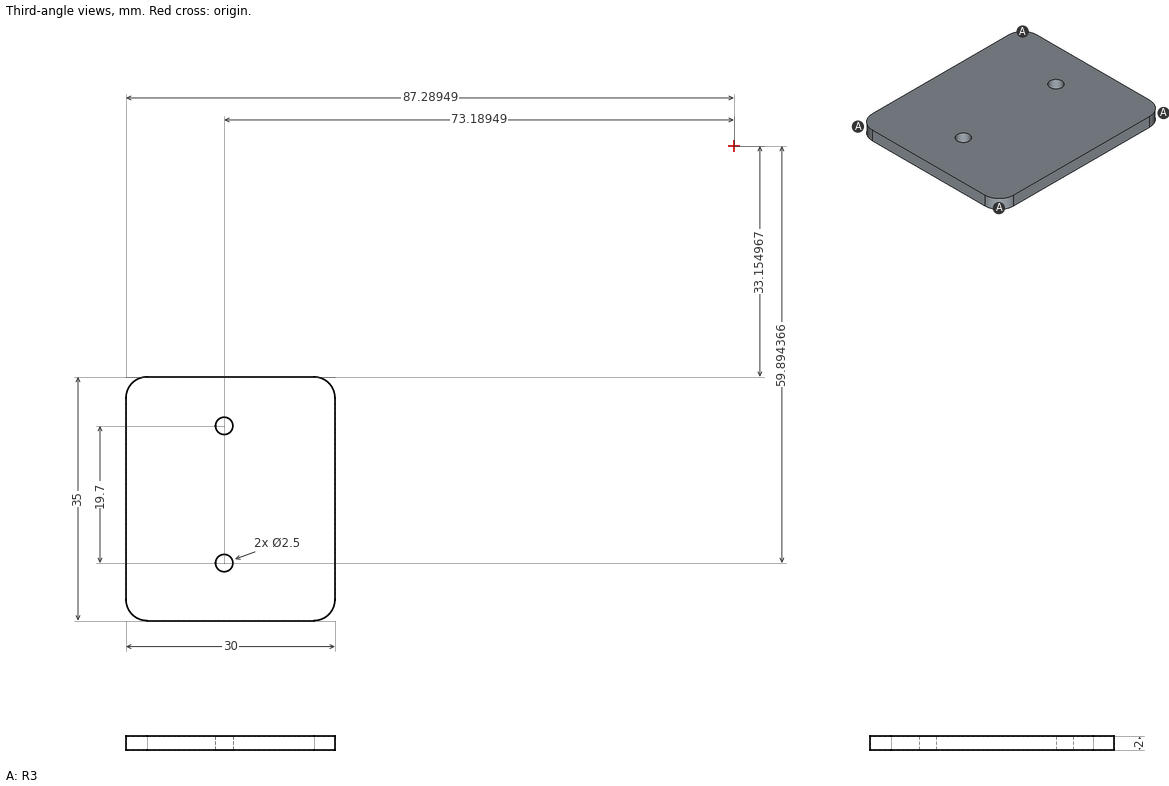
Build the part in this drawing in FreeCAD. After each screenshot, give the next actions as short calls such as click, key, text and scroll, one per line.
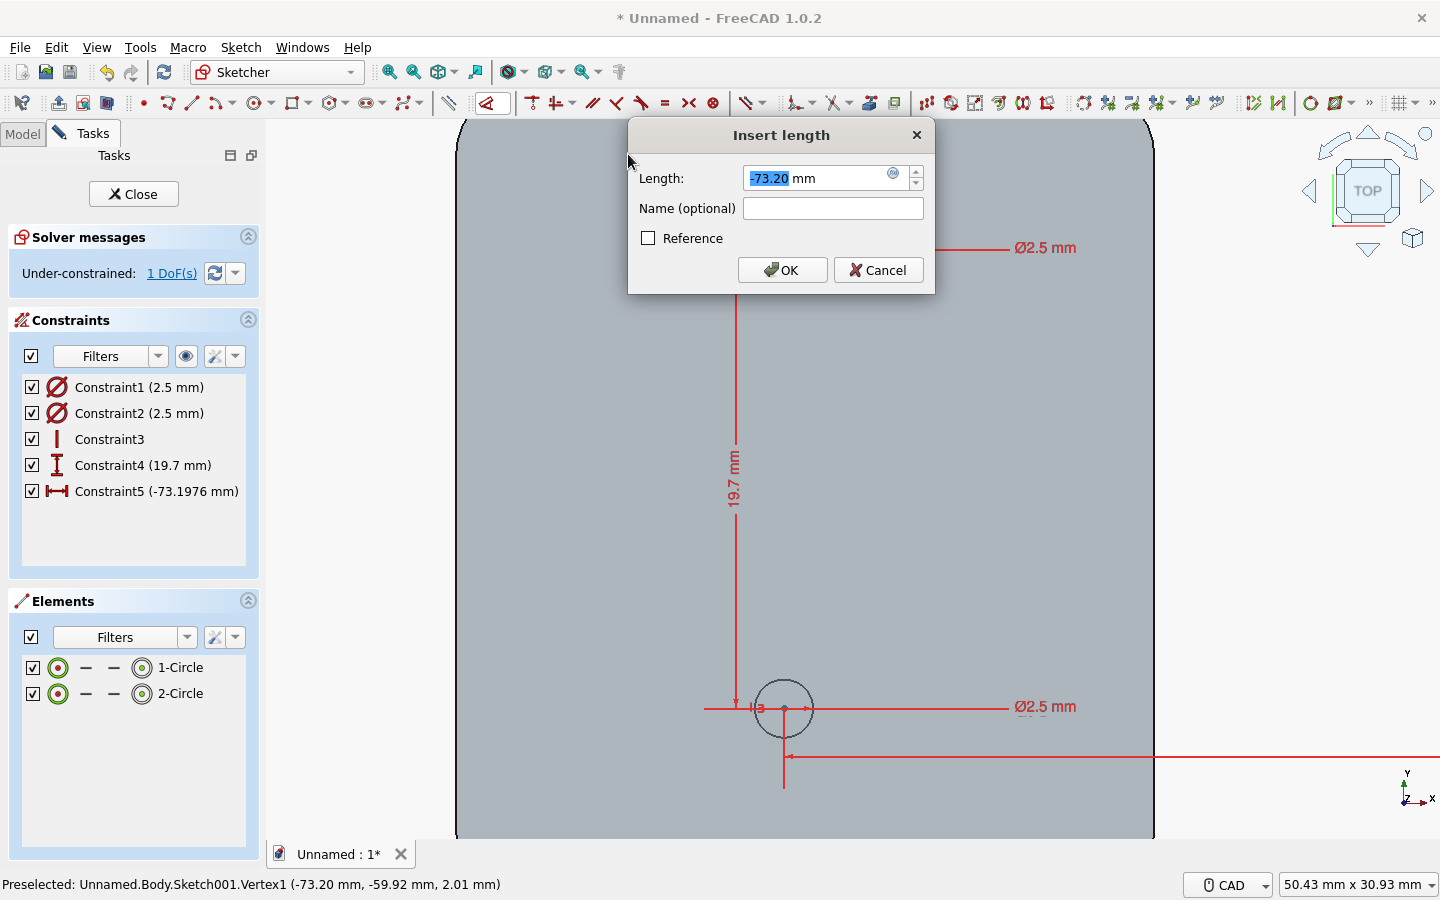
text(-73.18949)
key(Return)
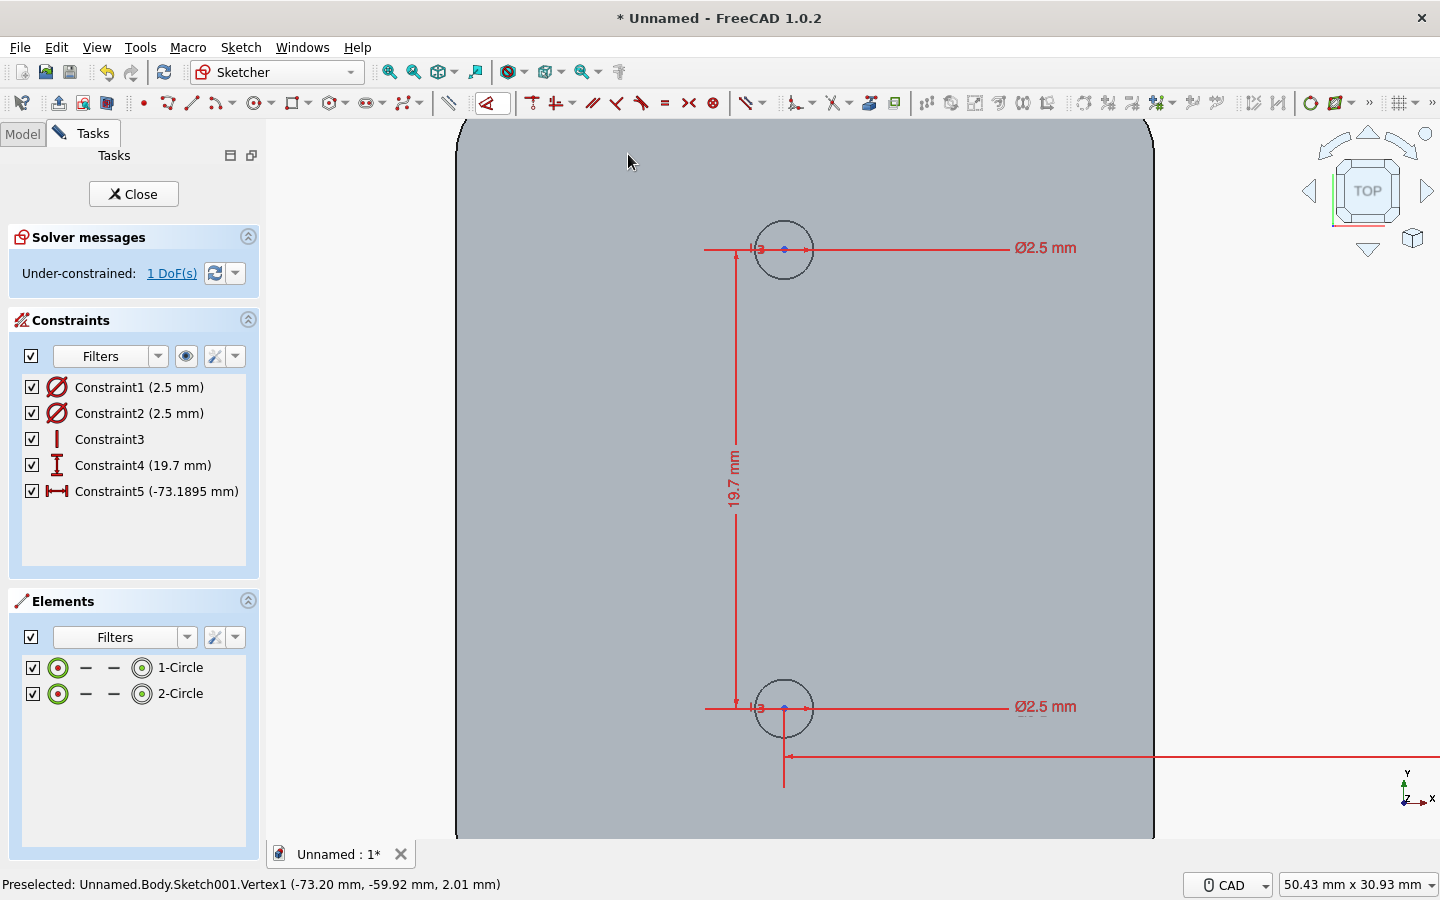
click(784, 709)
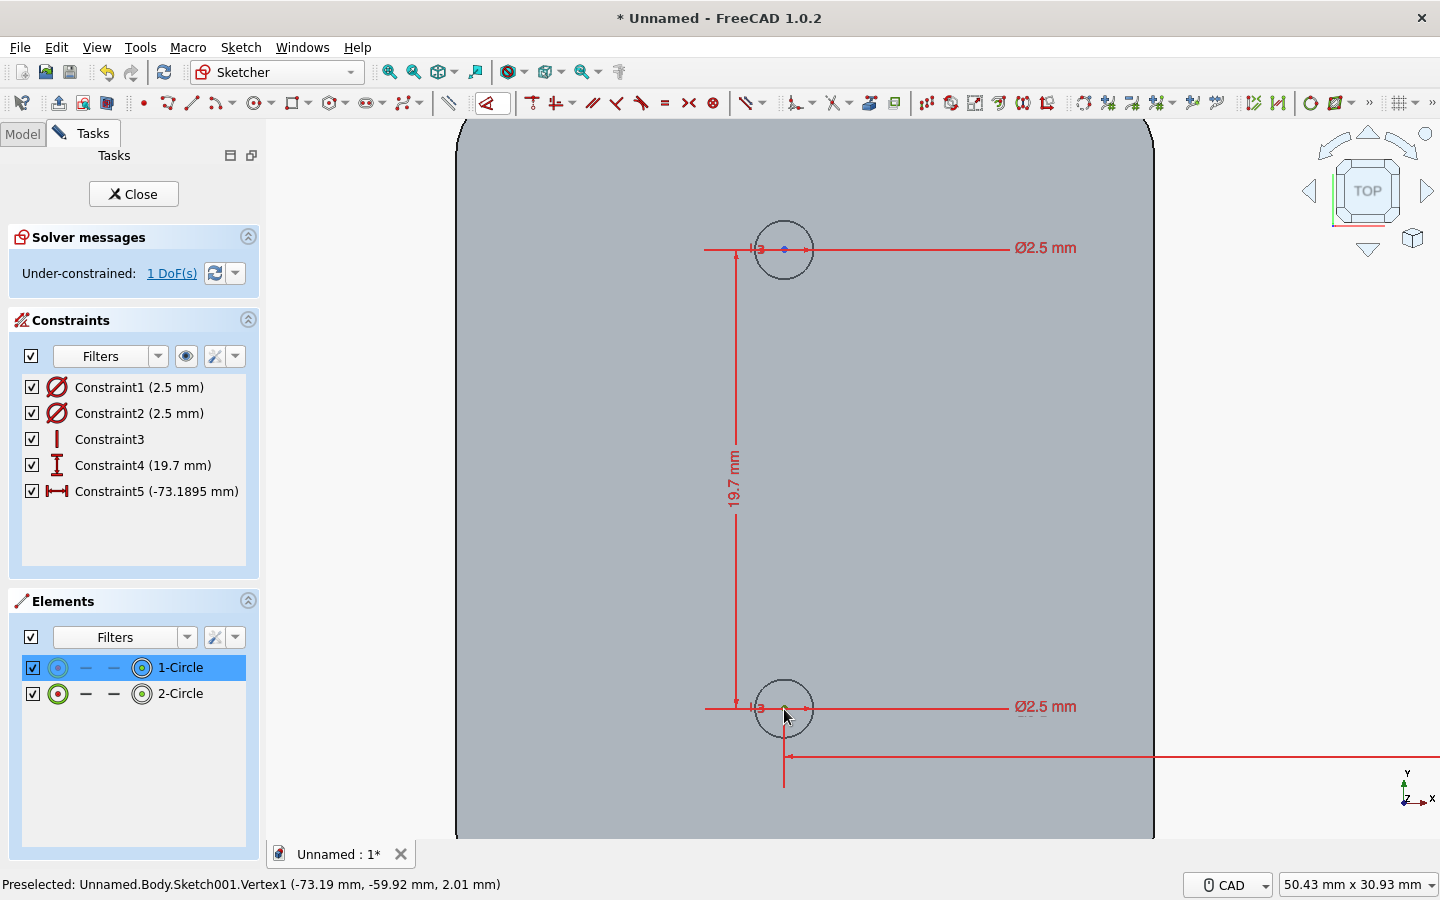
key(i)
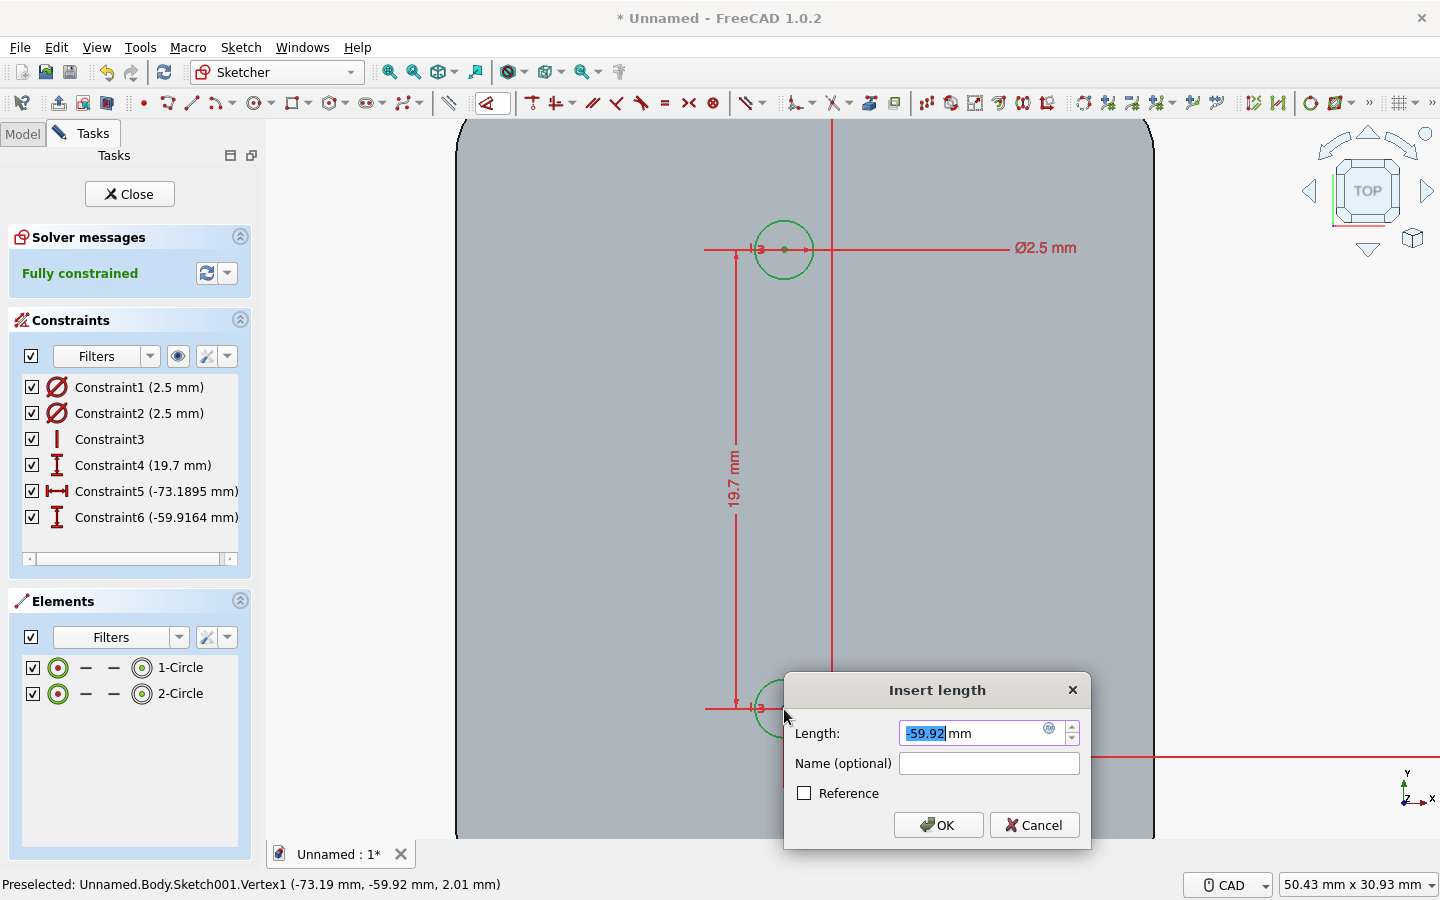
text(-59.894366)
key(Return)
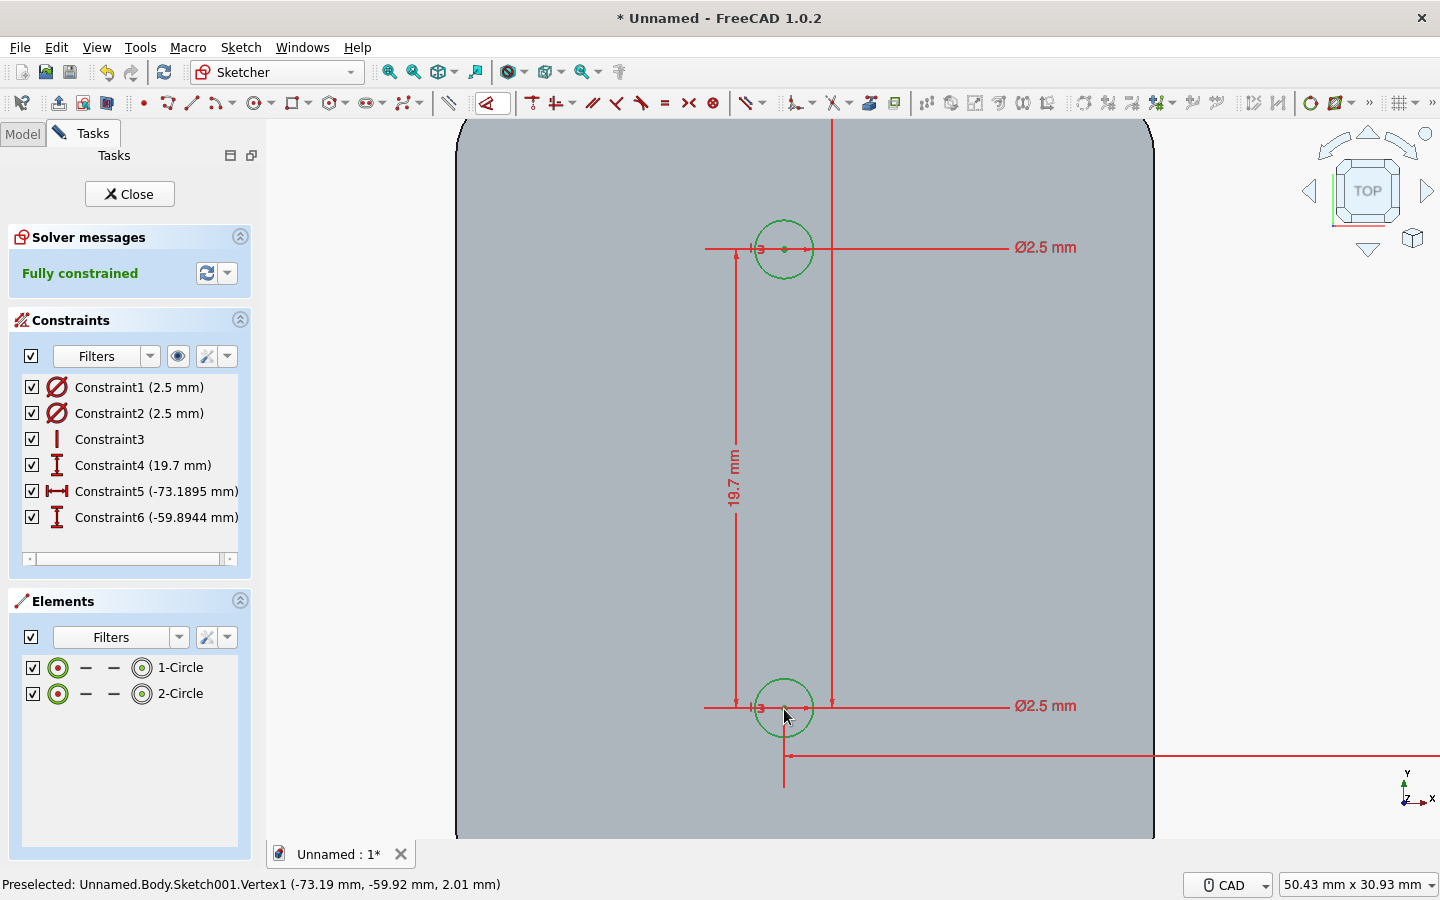
click(130, 194)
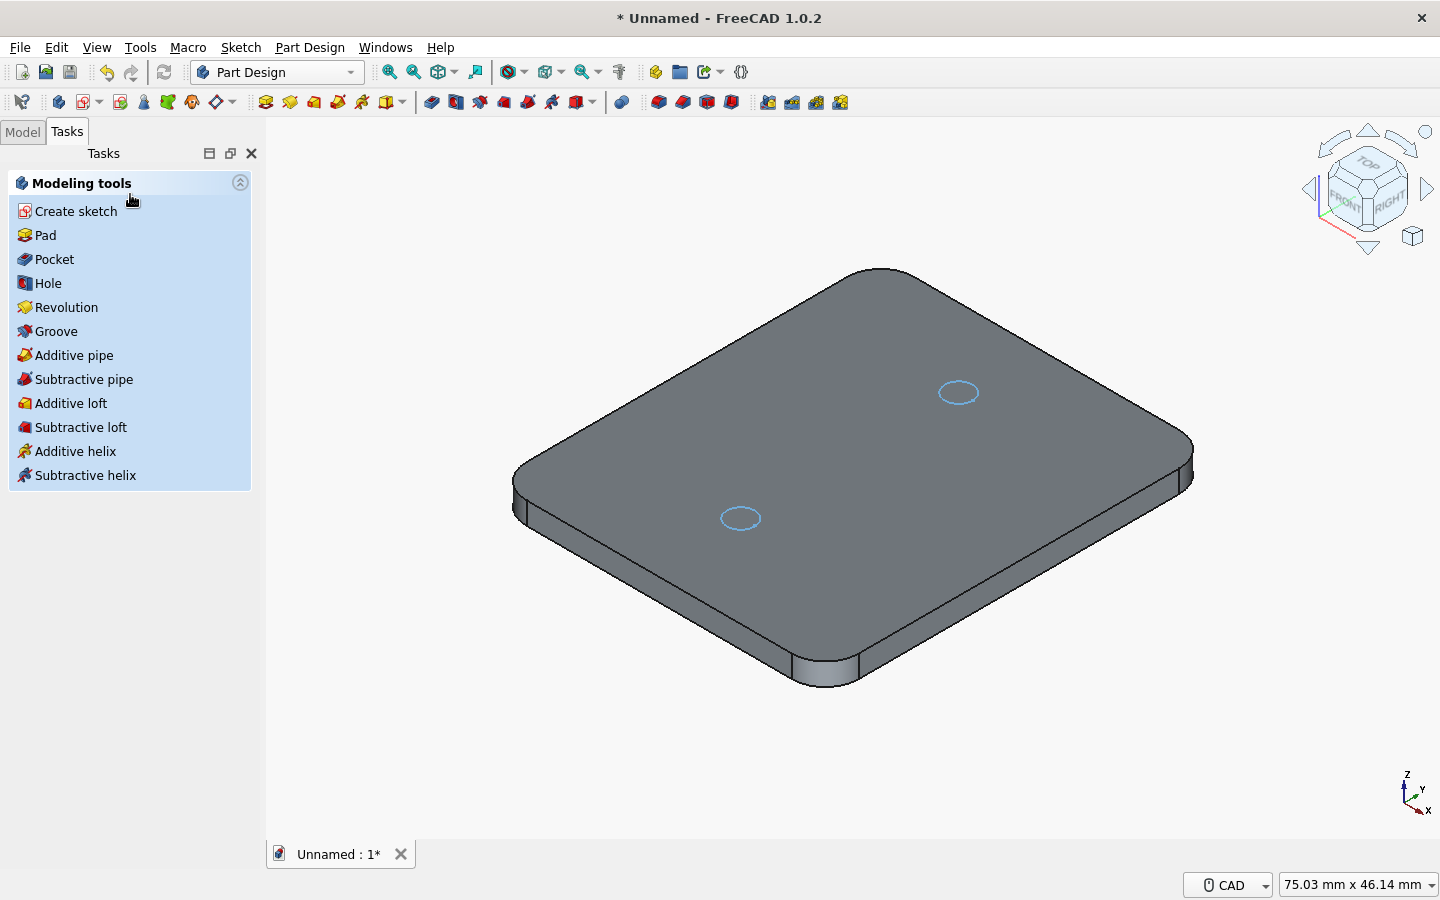
click(432, 102)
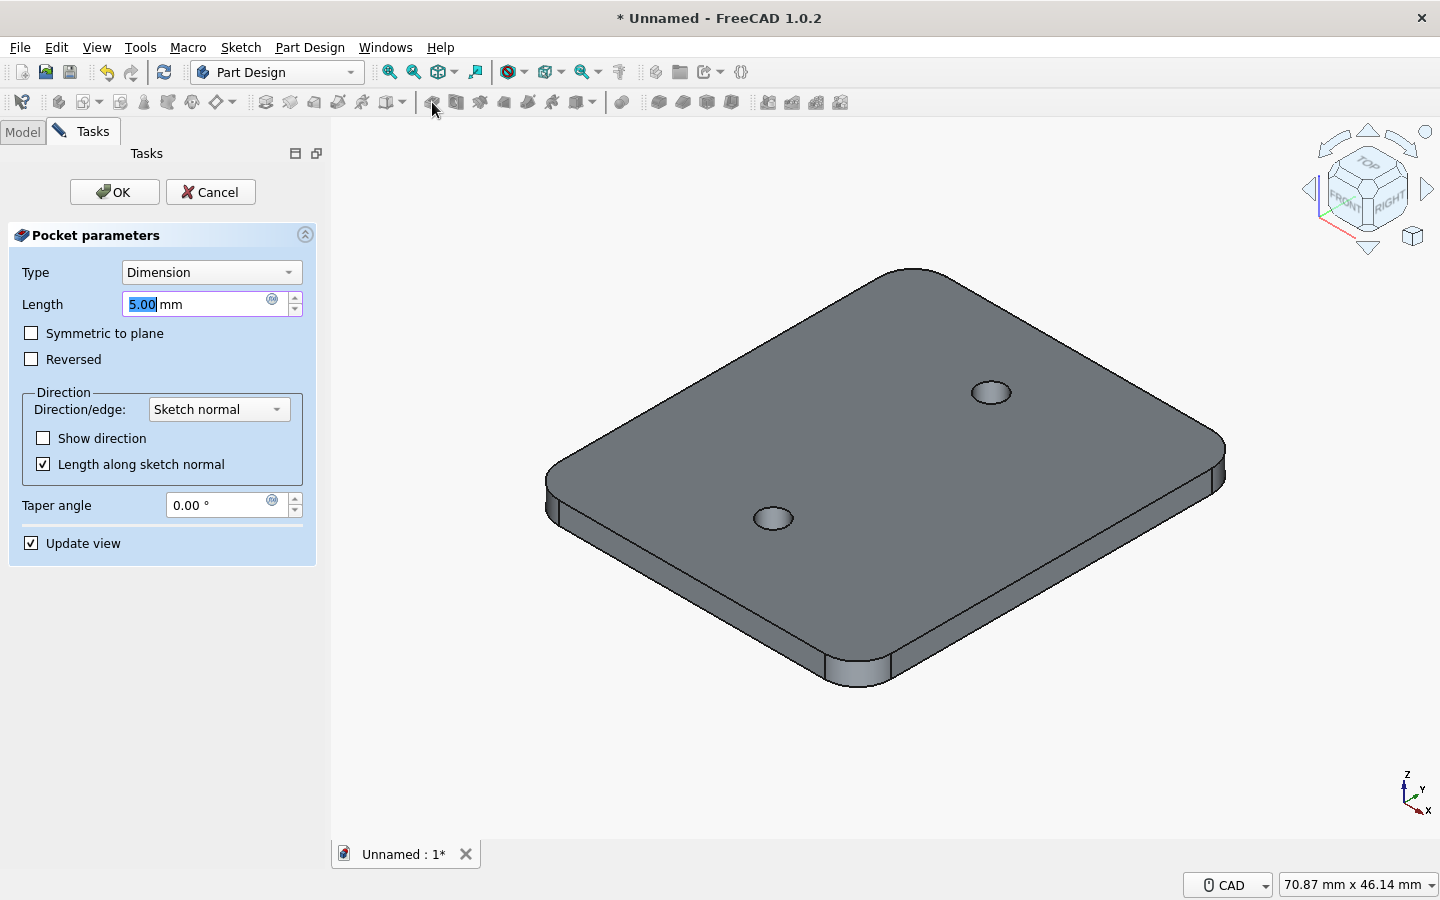
click(212, 272)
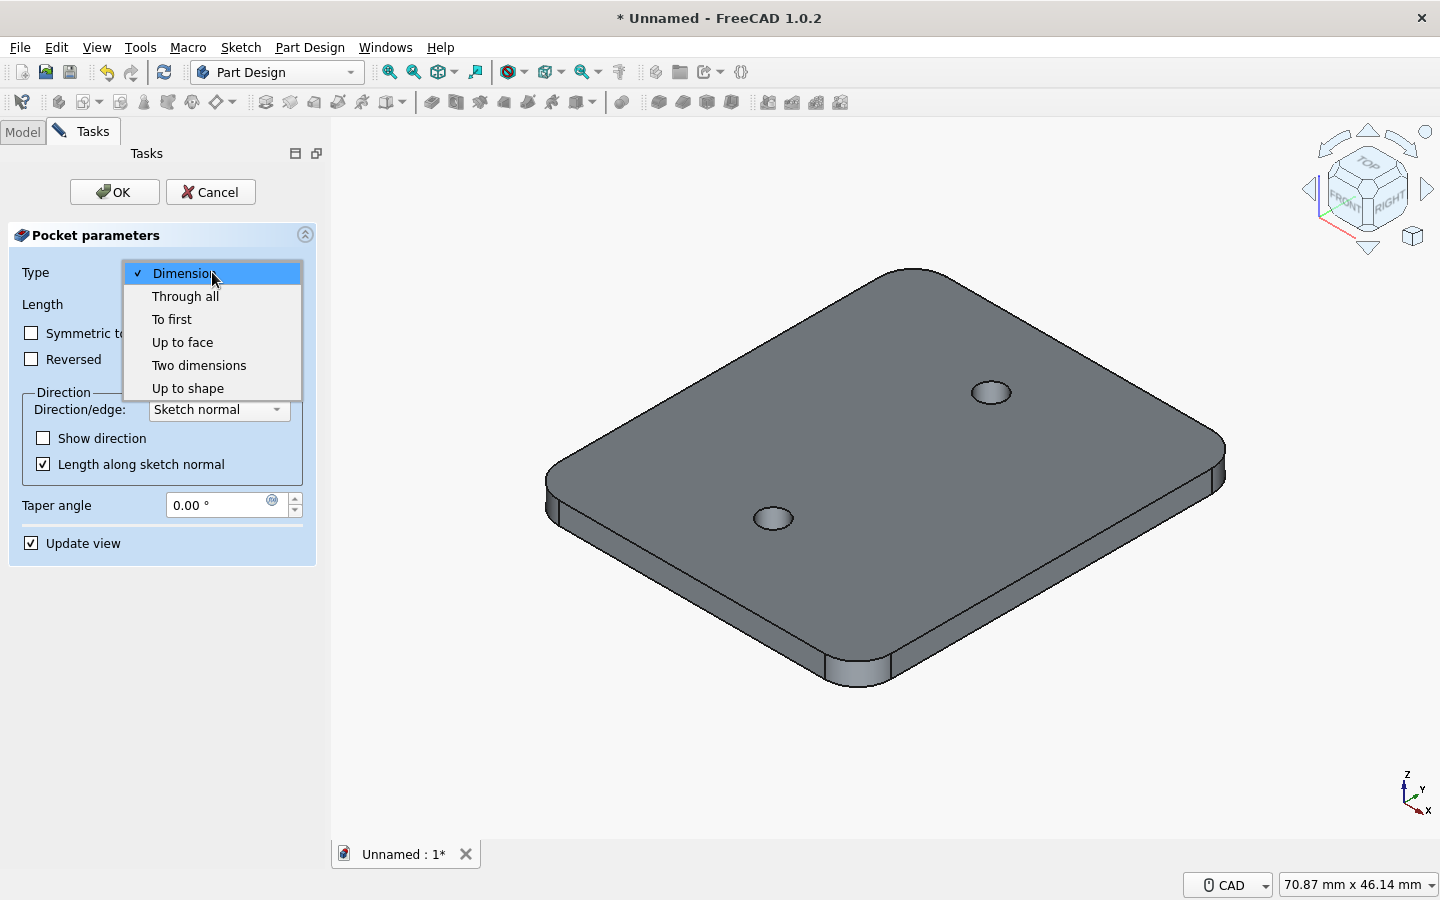
click(212, 296)